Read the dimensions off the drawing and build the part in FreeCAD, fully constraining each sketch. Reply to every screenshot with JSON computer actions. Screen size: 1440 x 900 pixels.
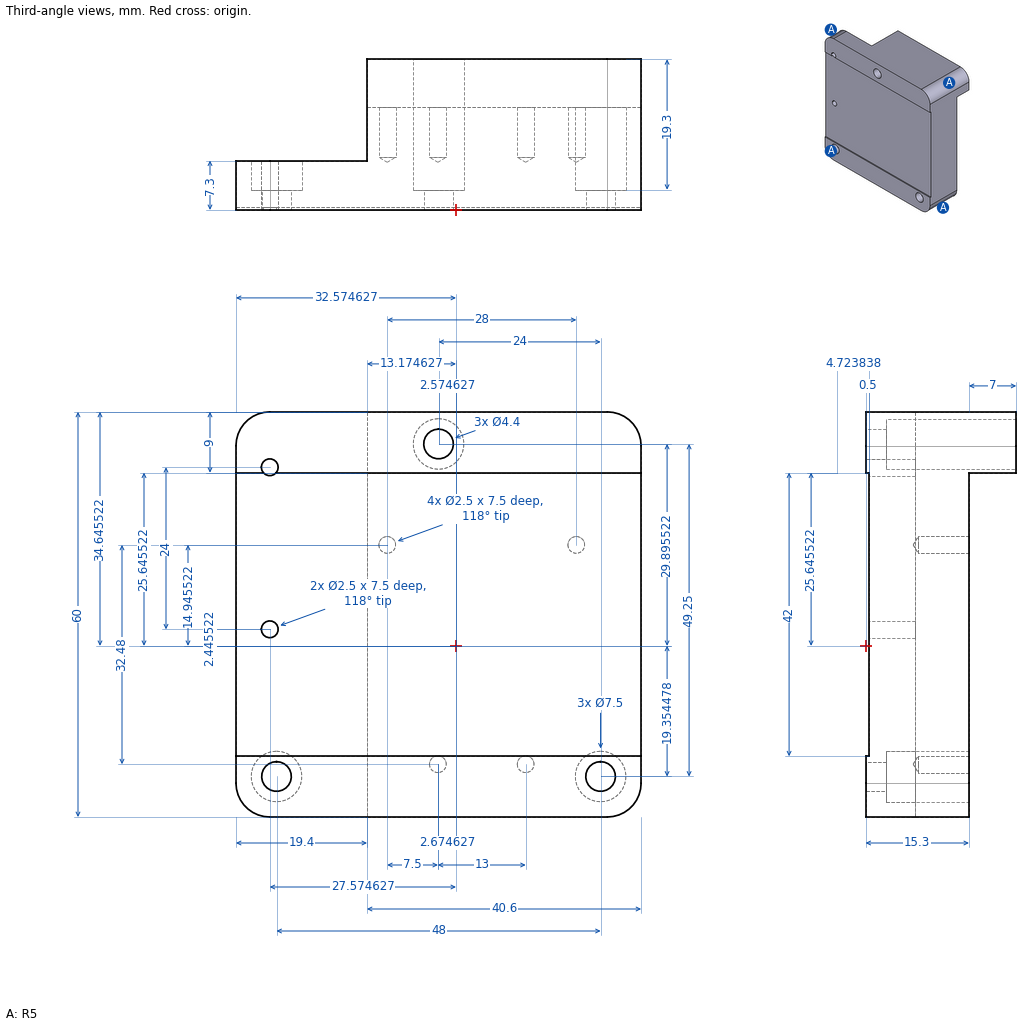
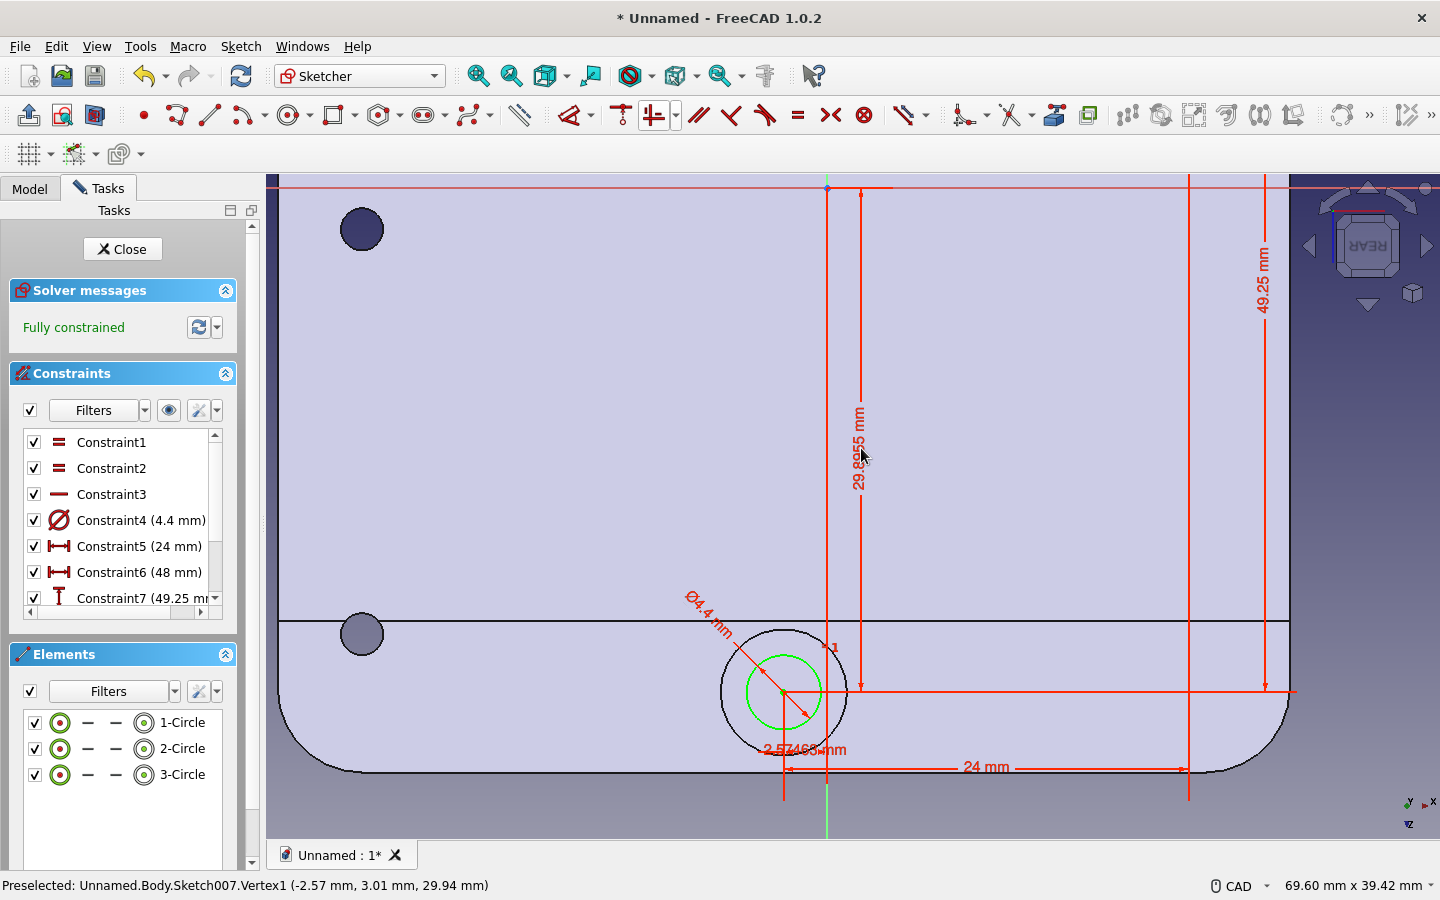
{"action": "left_click", "coordinate": [123, 249]}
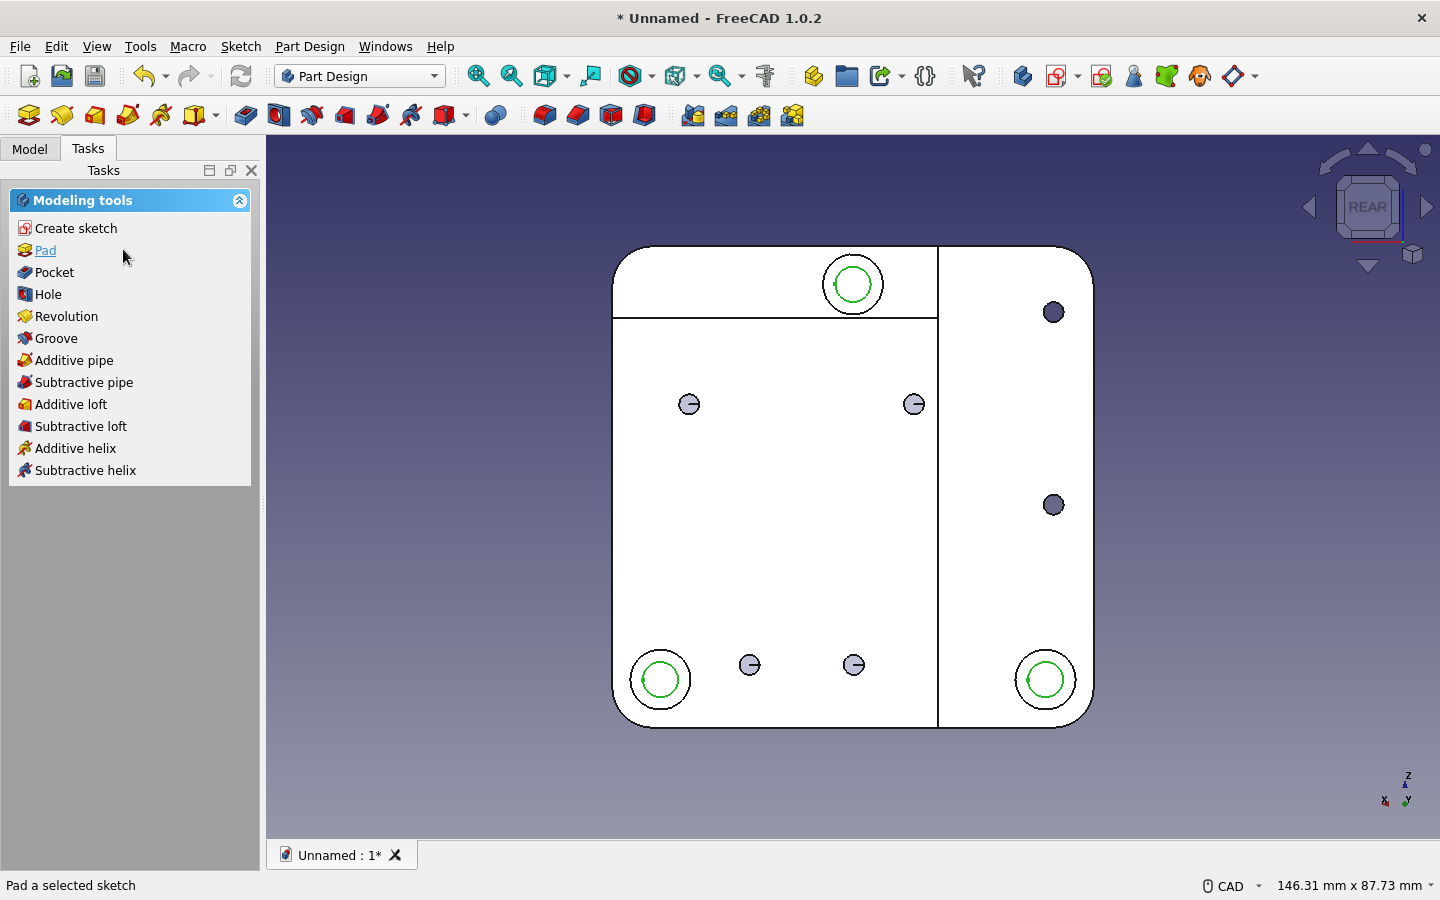
{"action": "left_click", "coordinate": [246, 116]}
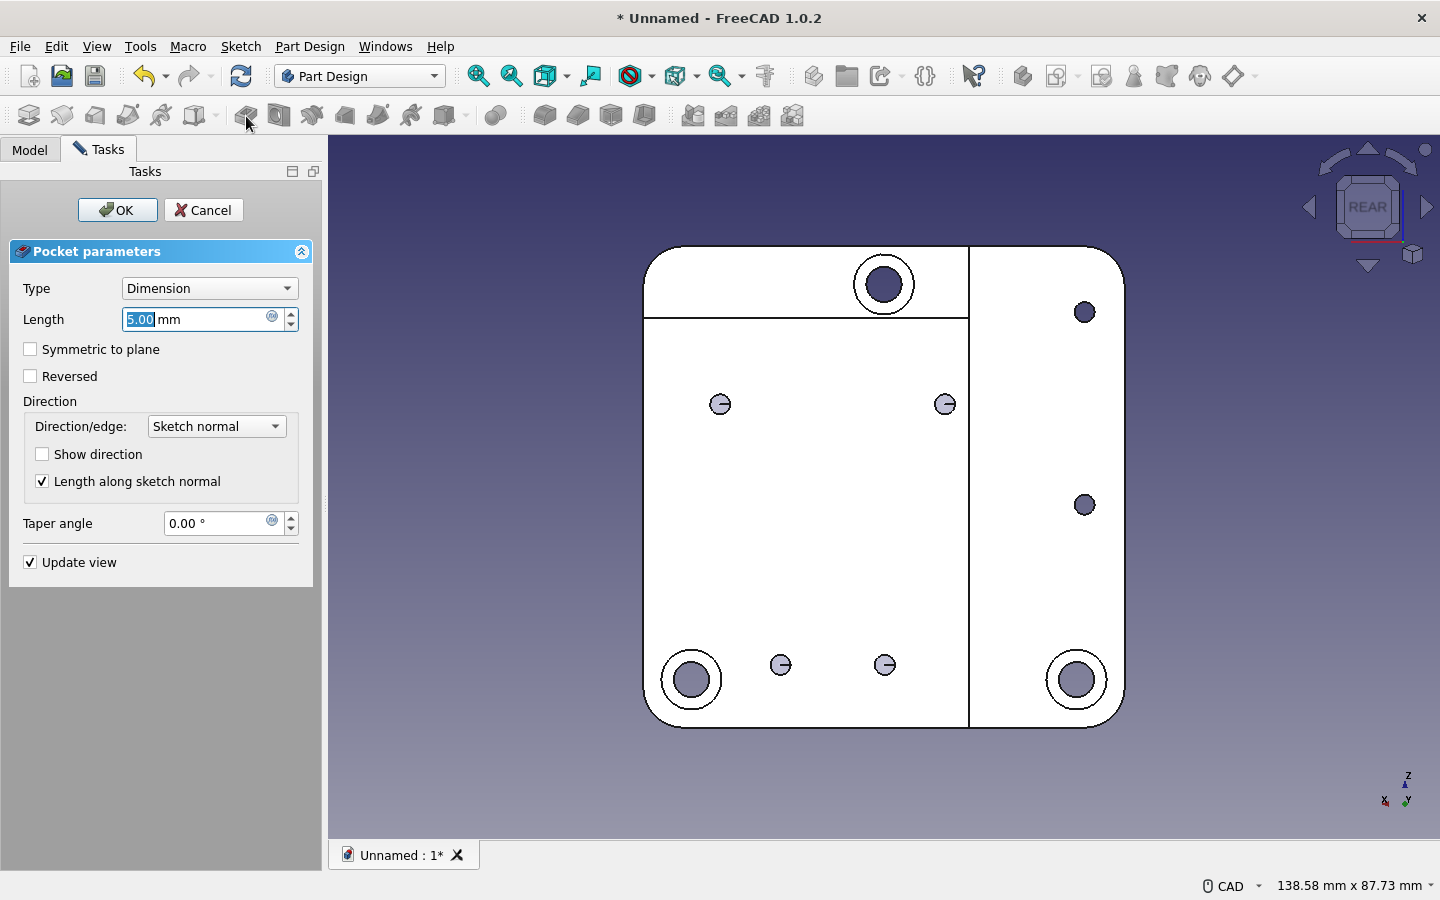
{"action": "left_click", "coordinate": [210, 288]}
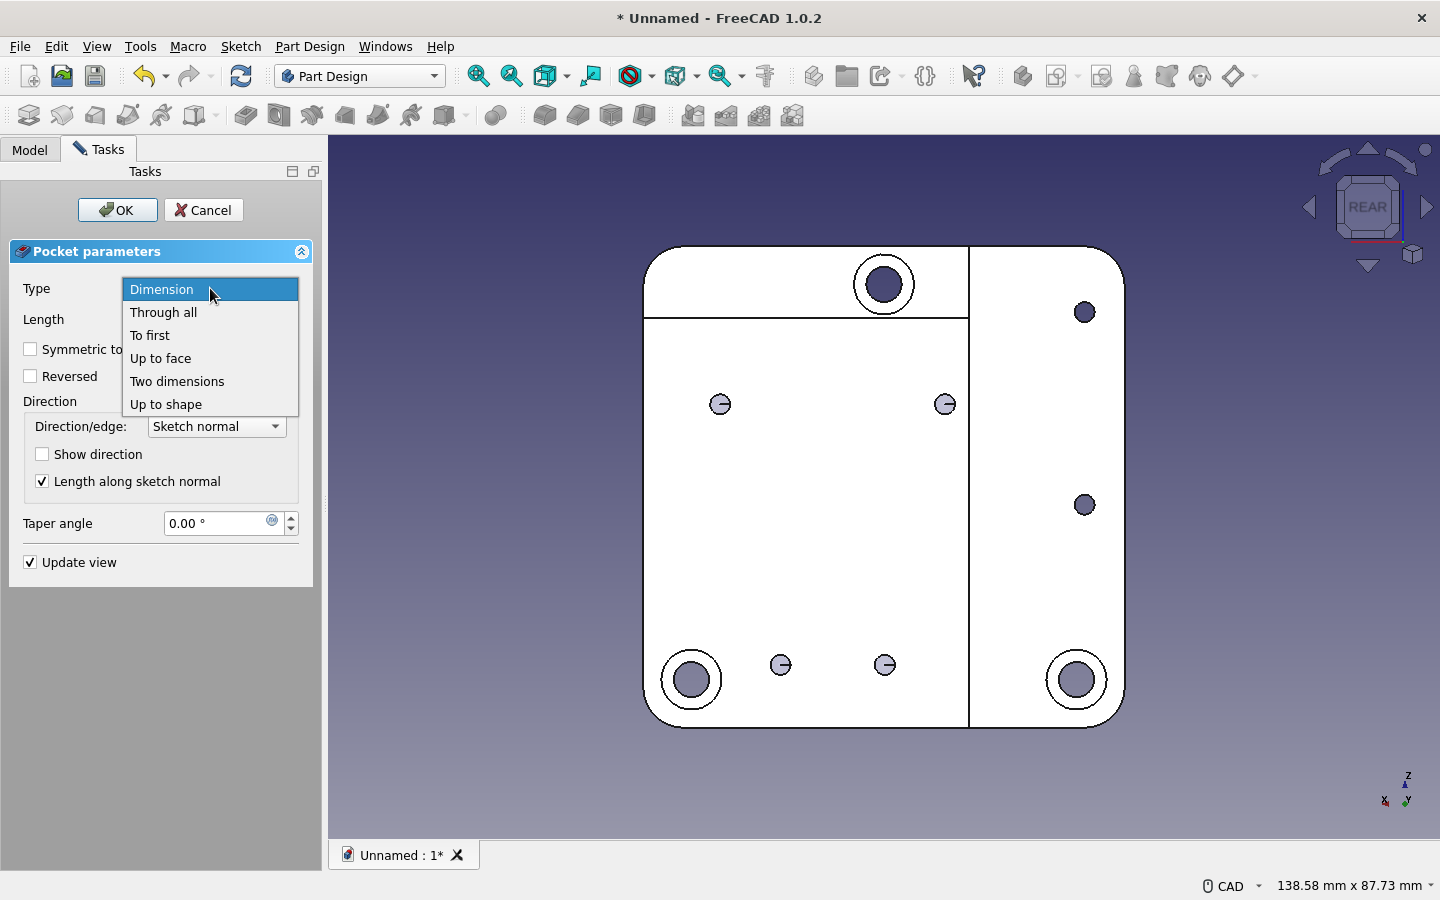
{"action": "left_click", "coordinate": [208, 312]}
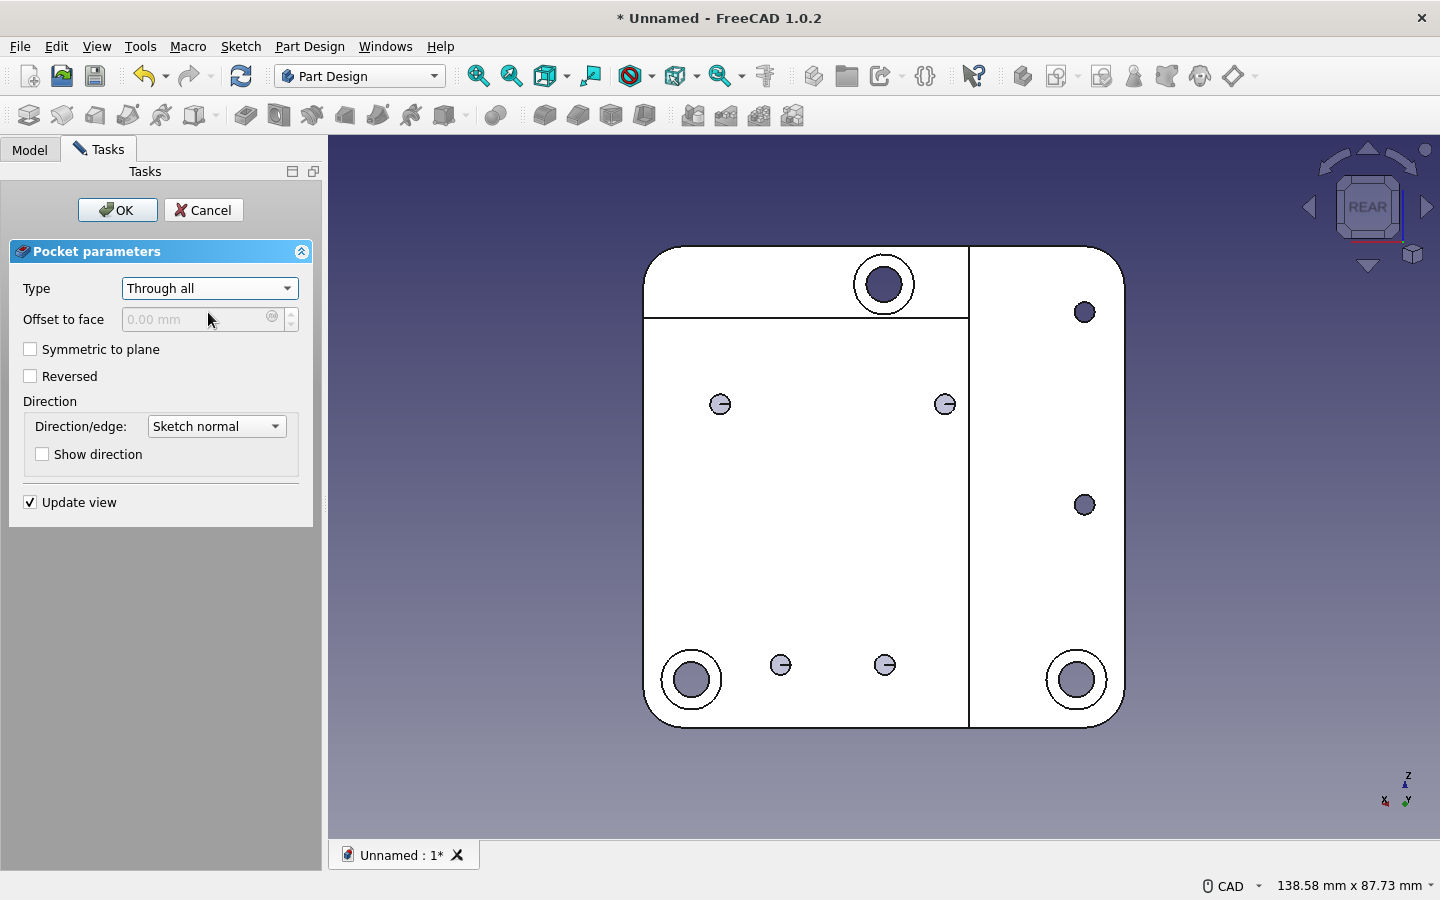
{"action": "left_click", "coordinate": [118, 210]}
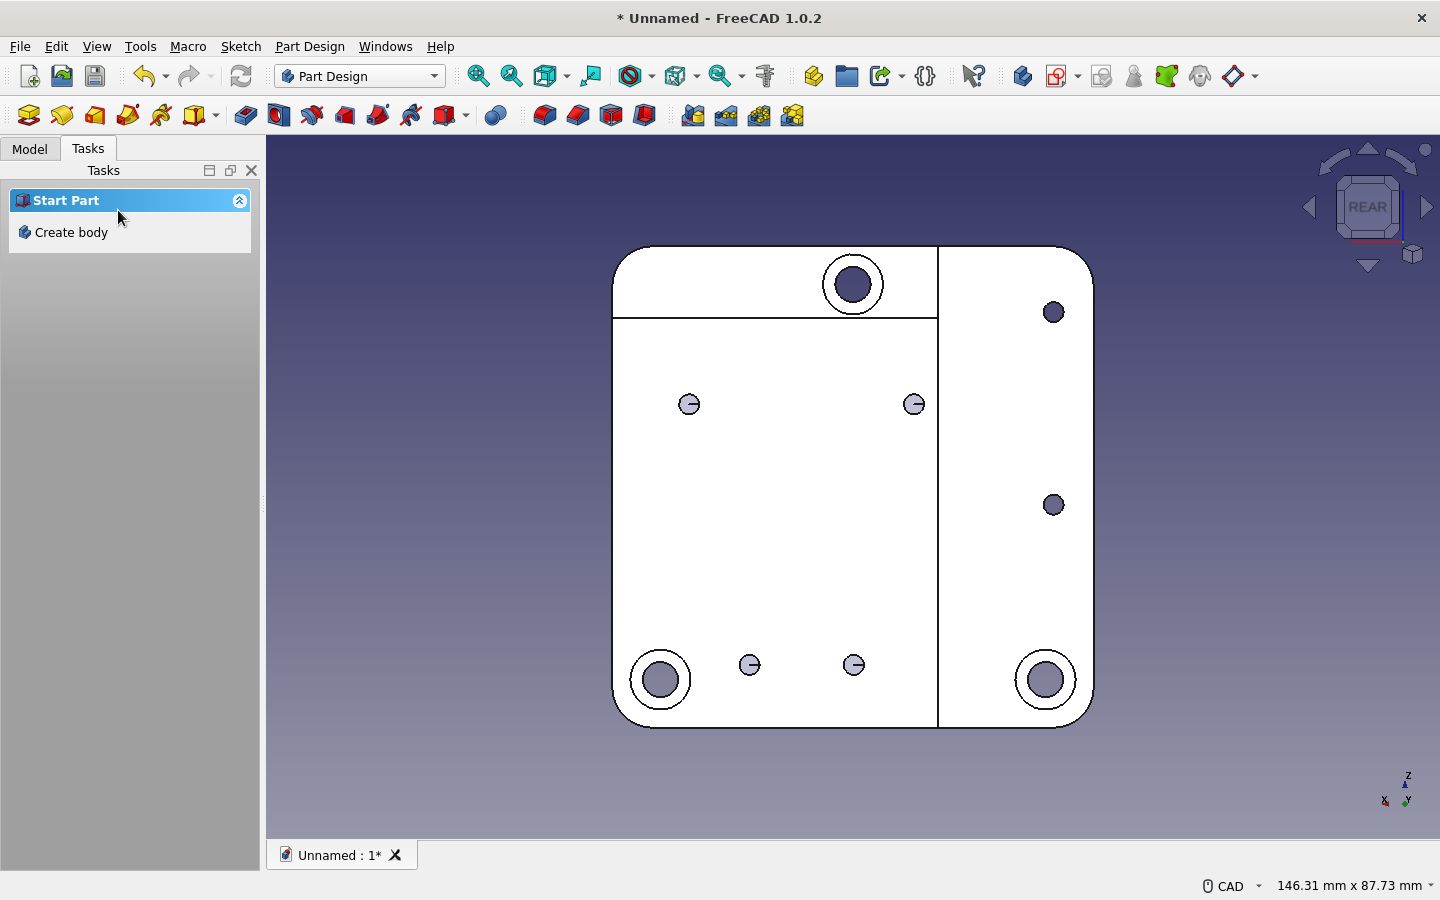
{"action": "key", "text": "0"}